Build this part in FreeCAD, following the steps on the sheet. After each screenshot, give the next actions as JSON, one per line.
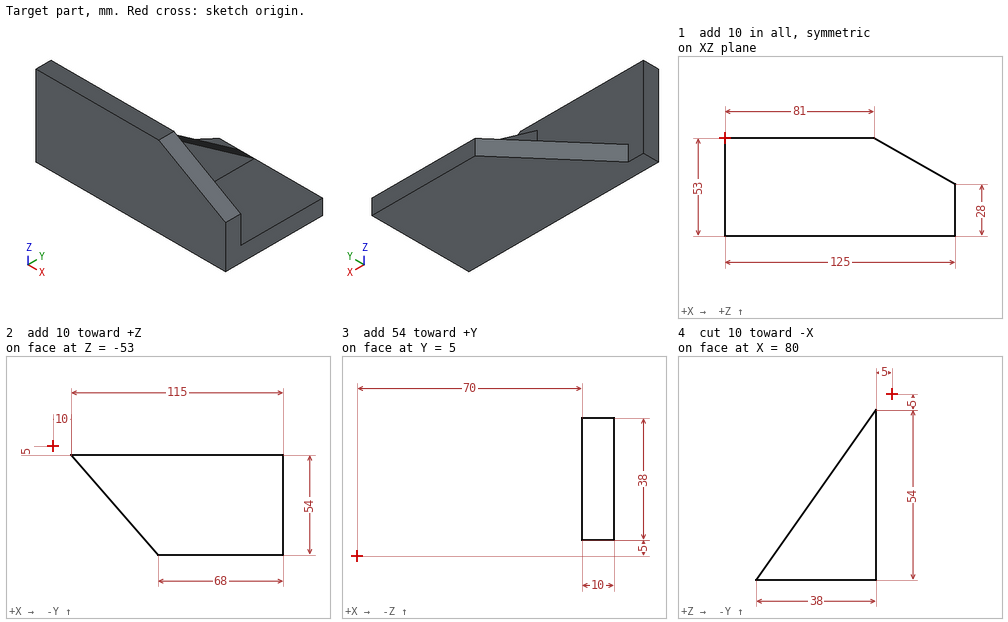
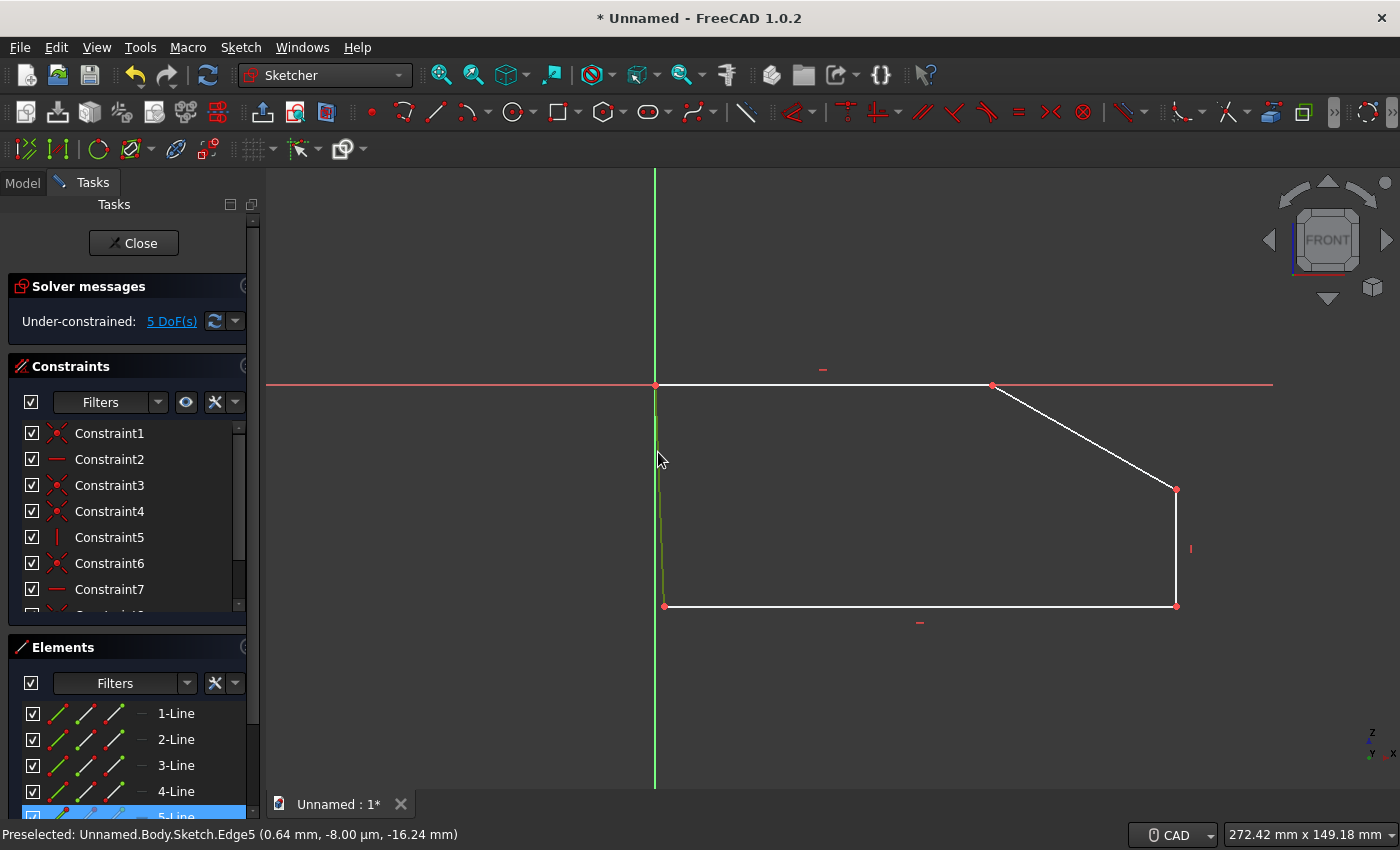
{"action": "key", "text": "v"}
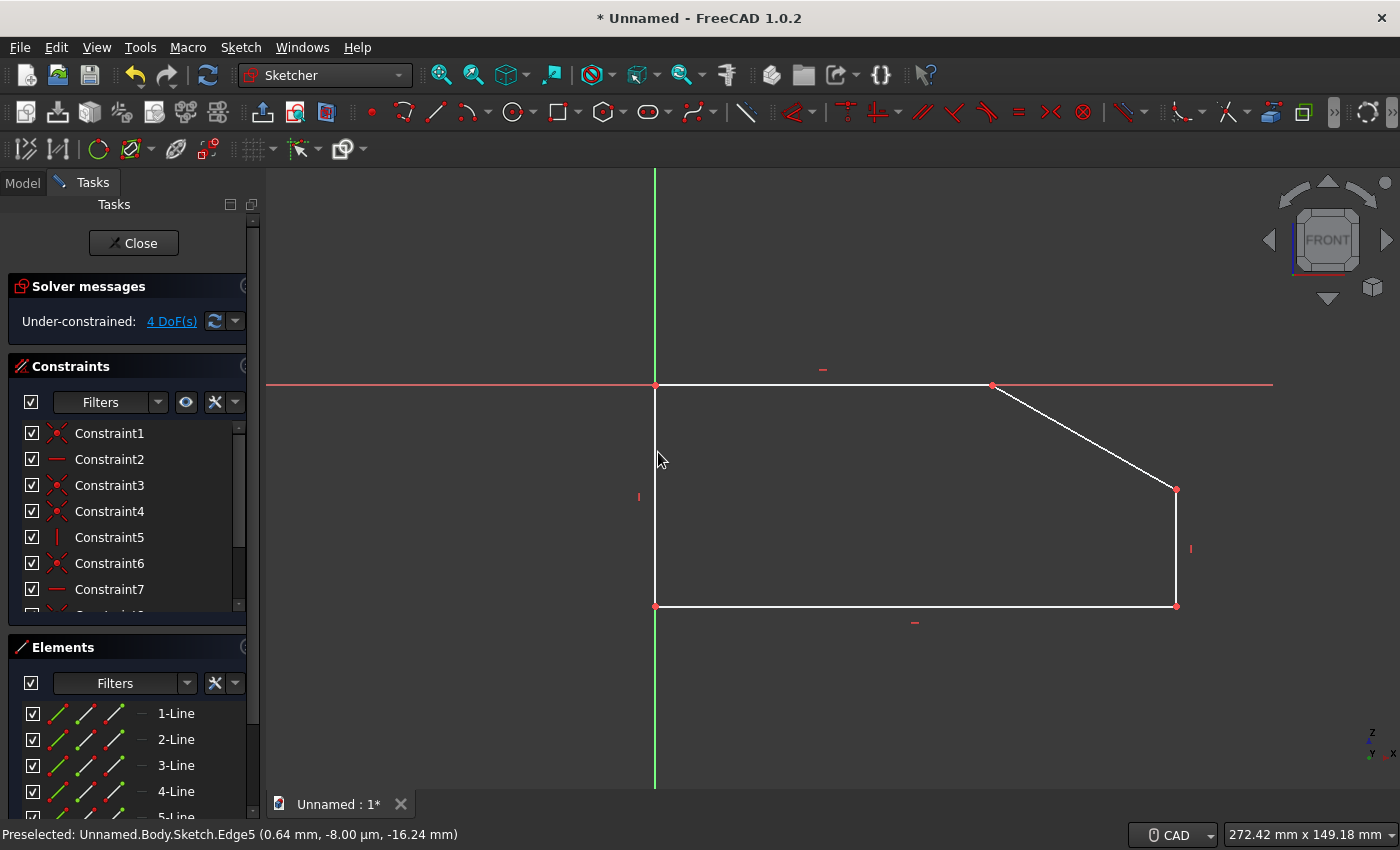
{"action": "left_click", "coordinate": [792, 112]}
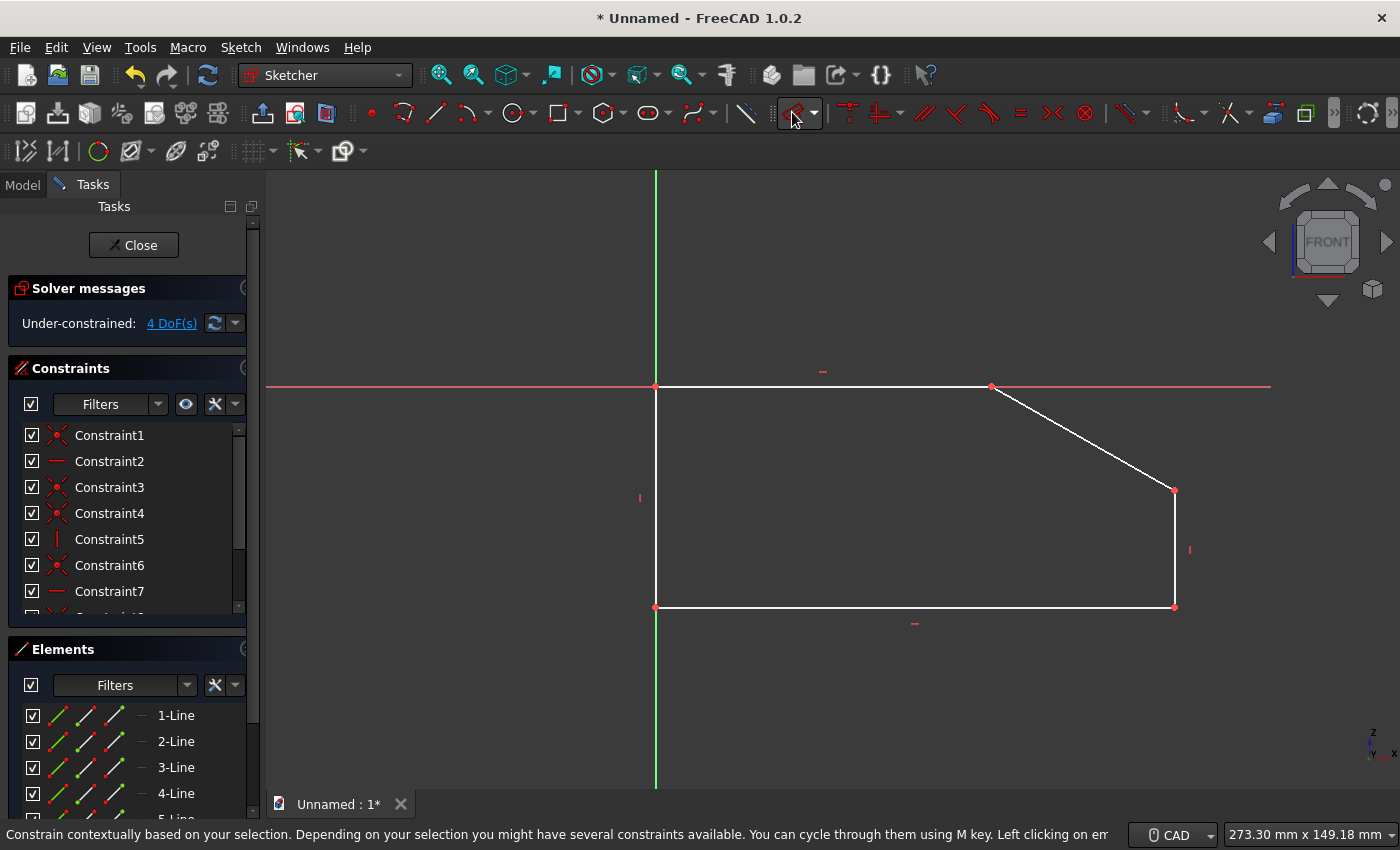
{"action": "left_click", "coordinate": [757, 387]}
{"action": "left_click", "coordinate": [824, 353]}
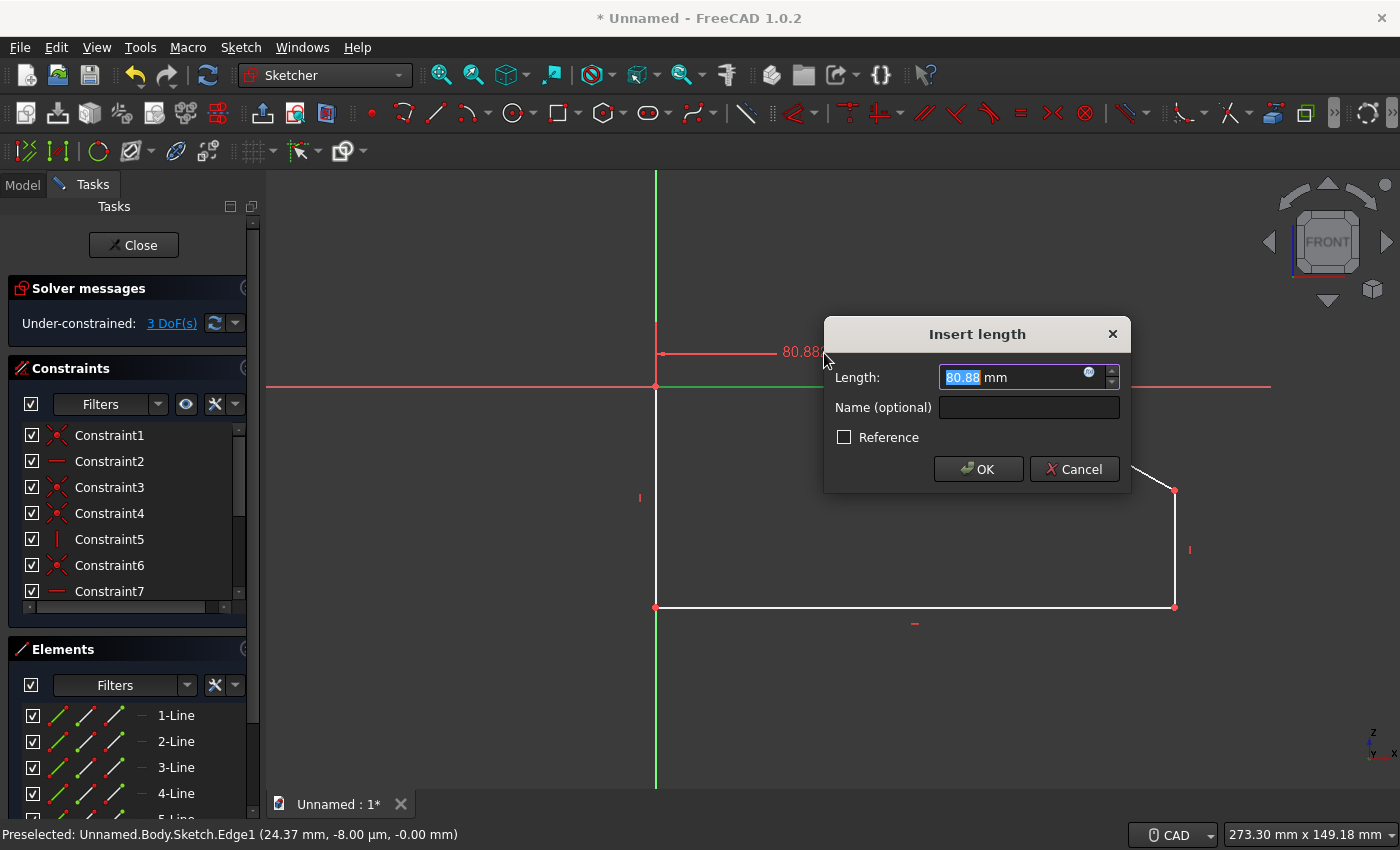
{"action": "type", "text": "81"}
{"action": "key", "text": "Return"}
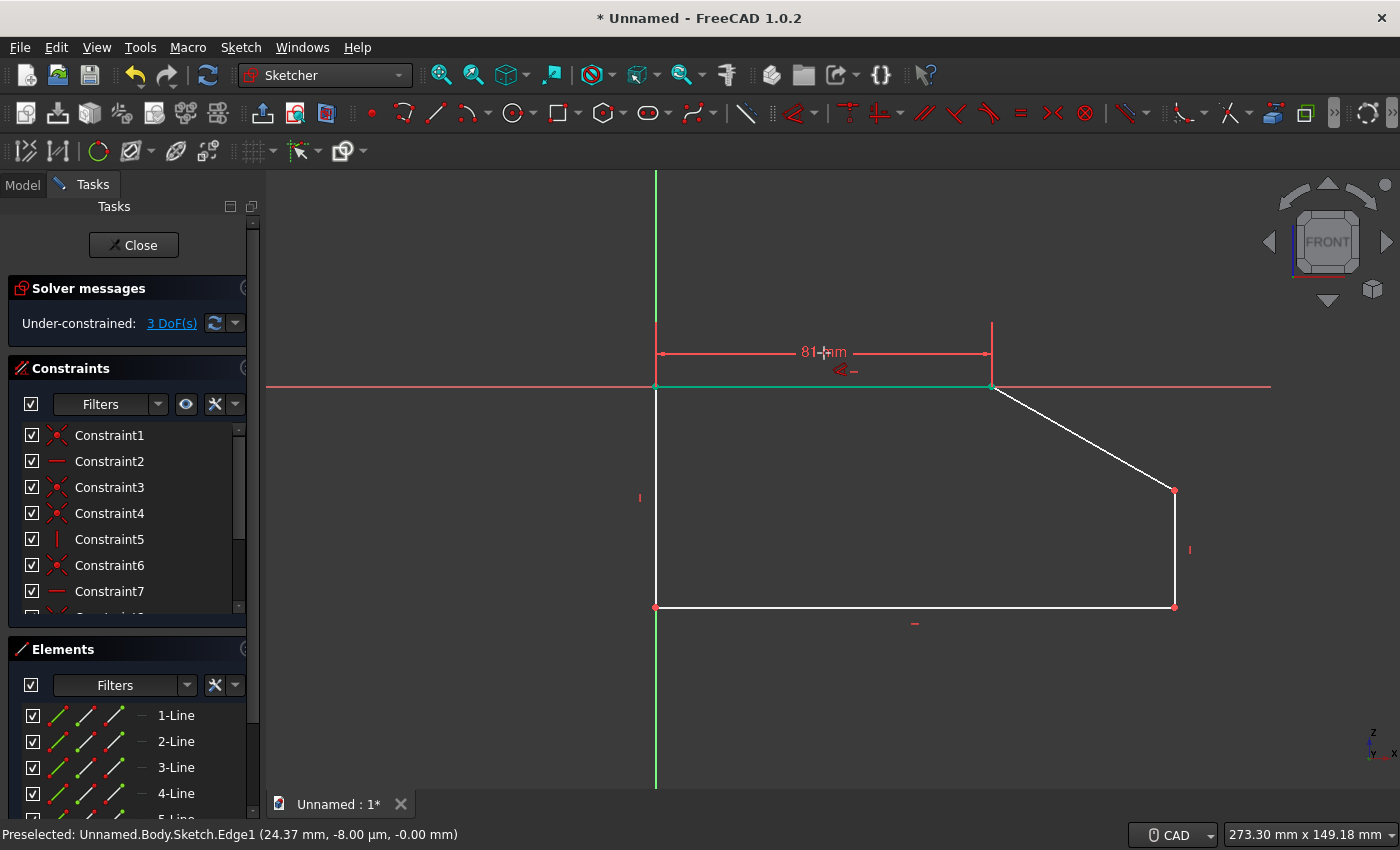
{"action": "left_click", "coordinate": [1175, 526]}
{"action": "left_click", "coordinate": [1209, 549]}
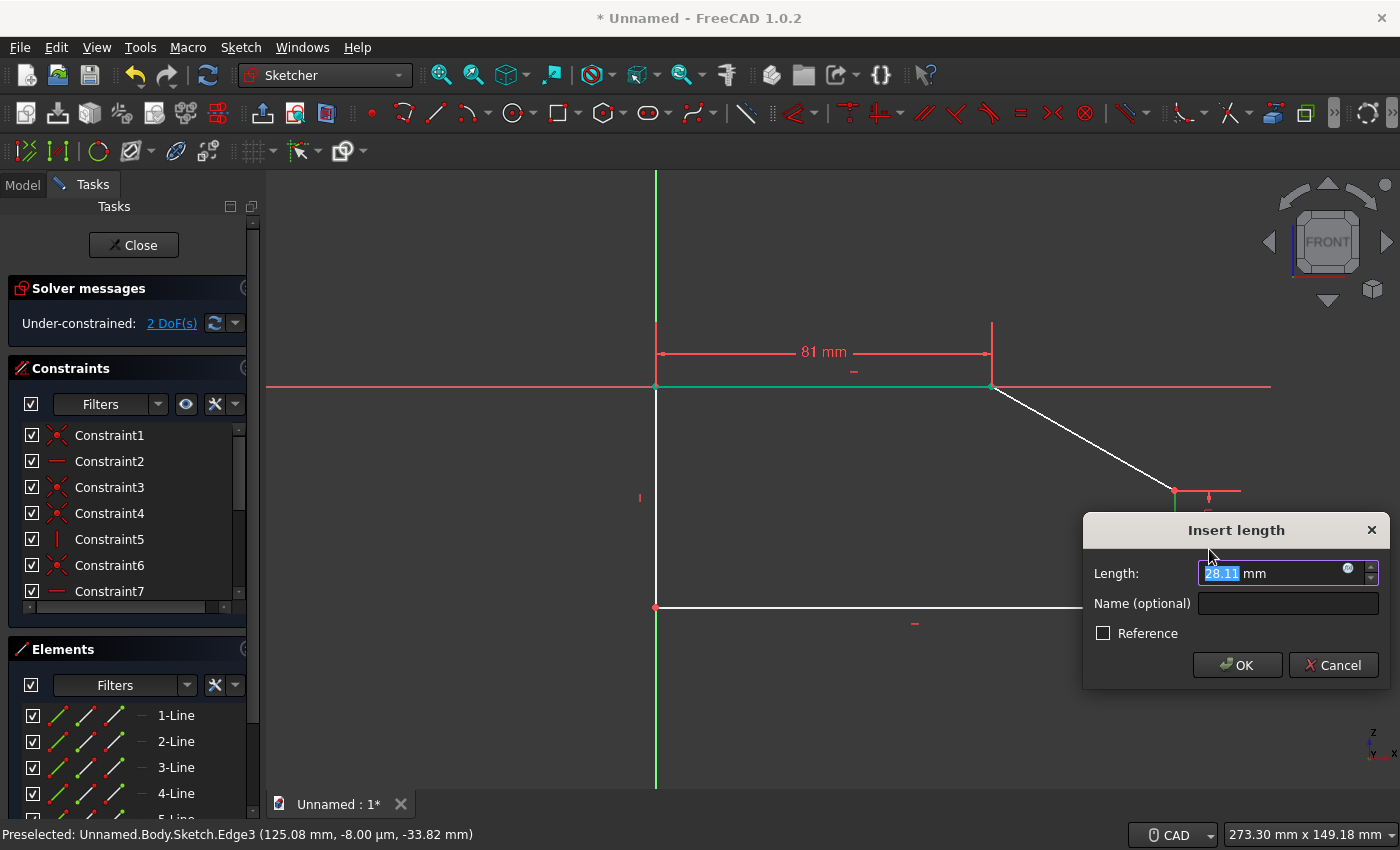
{"action": "type", "text": "28"}
{"action": "key", "text": "Return"}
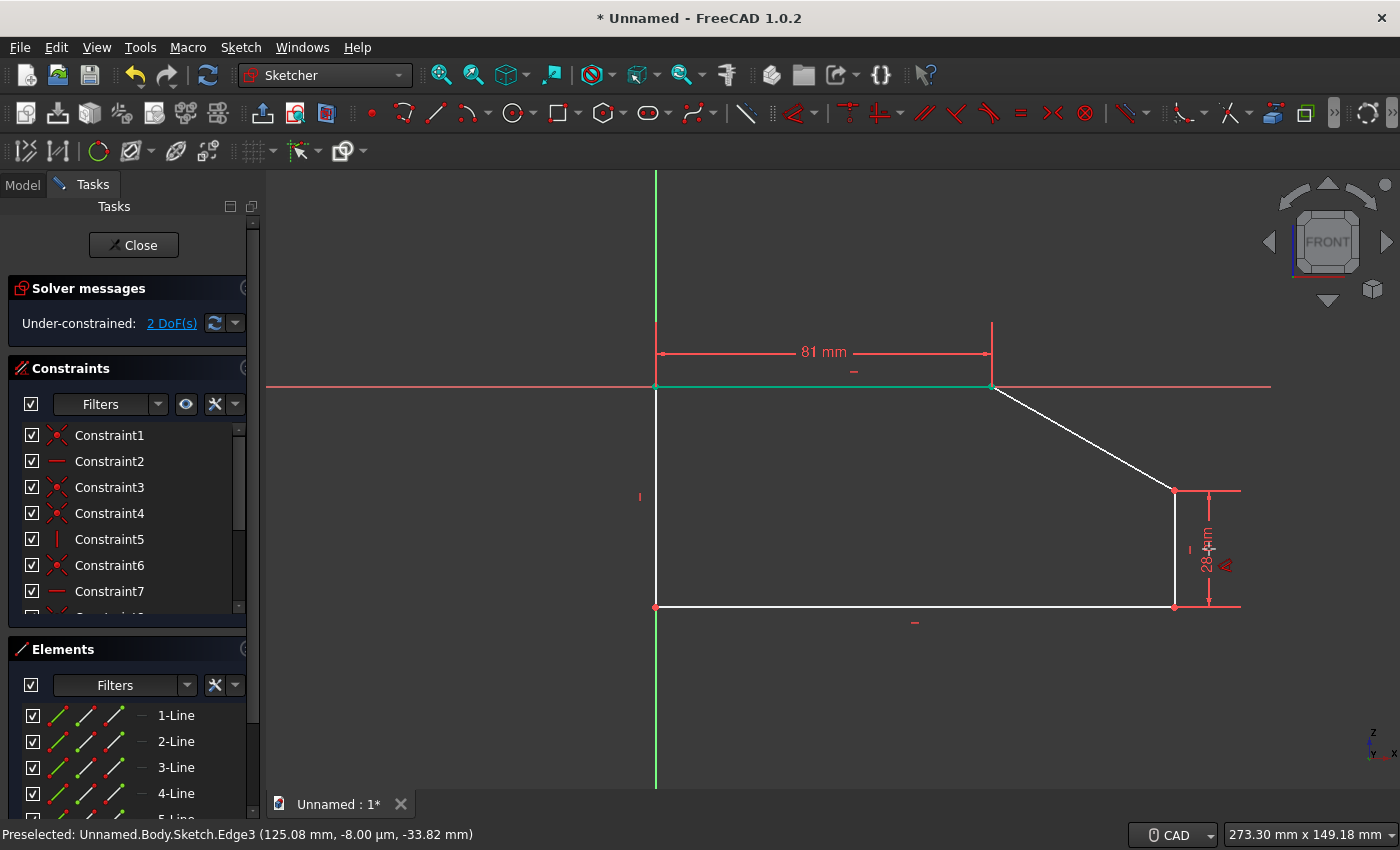
{"action": "left_click", "coordinate": [656, 541]}
{"action": "left_click", "coordinate": [622, 497]}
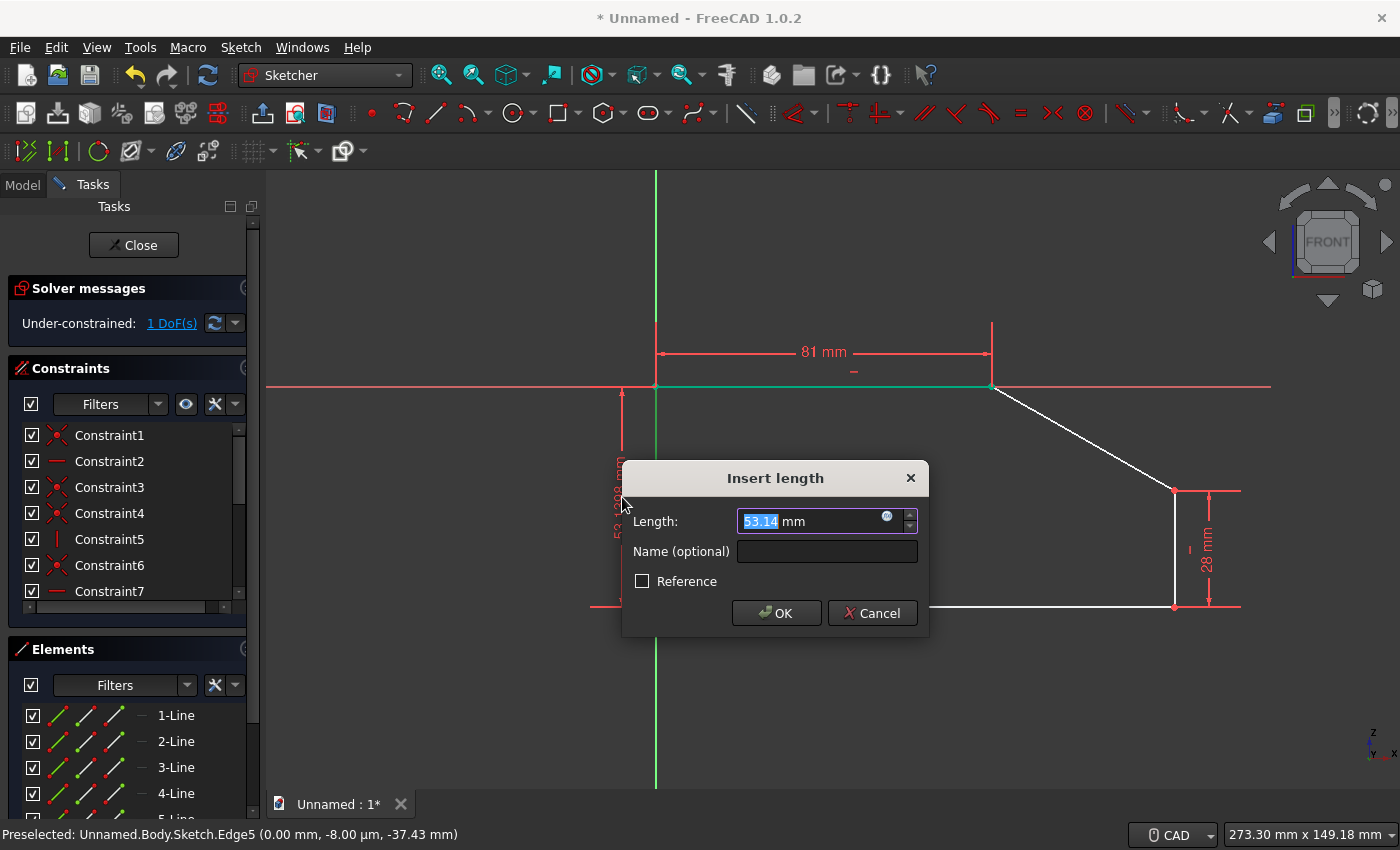
{"action": "type", "text": "53"}
{"action": "key", "text": "Return"}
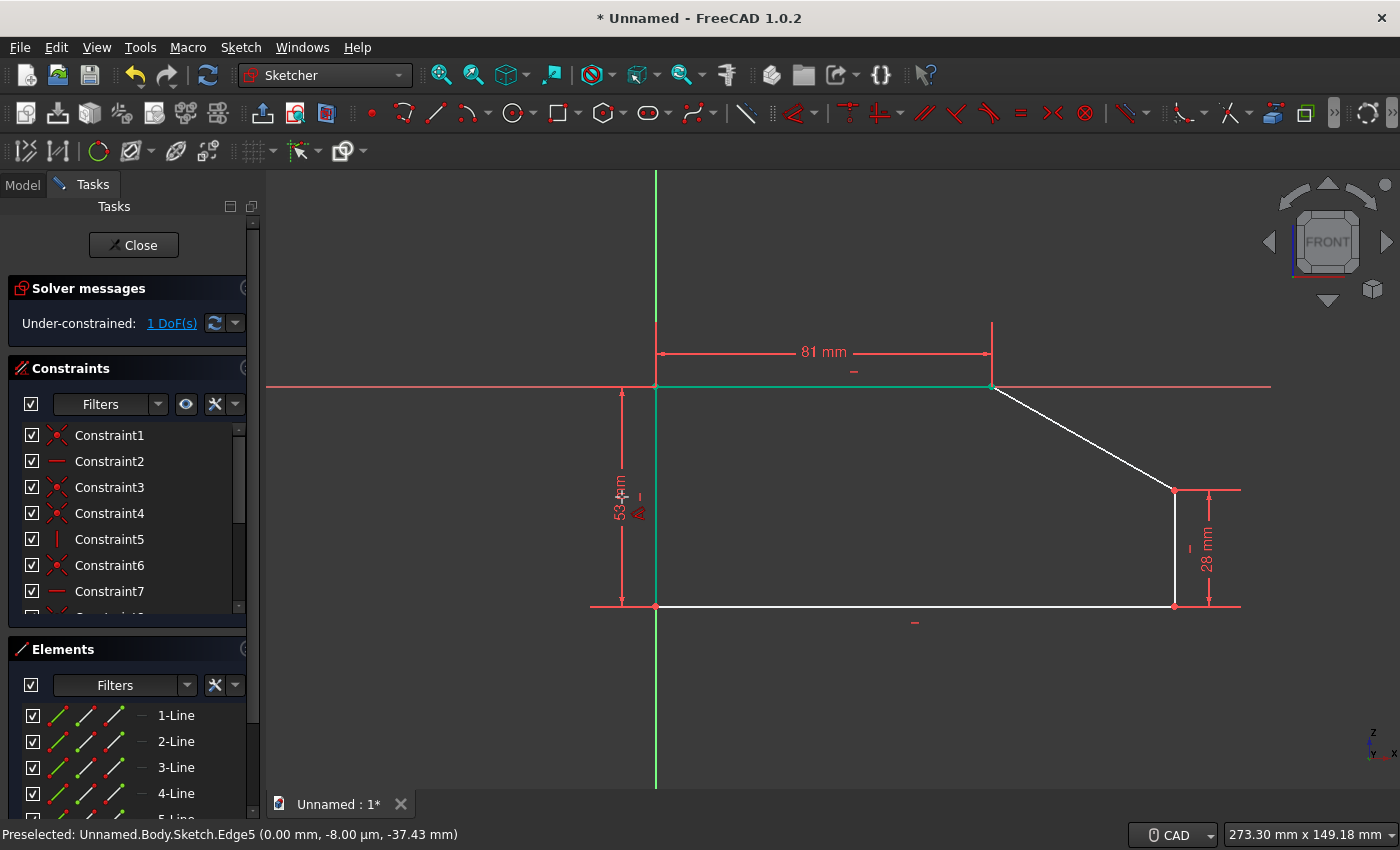
{"action": "left_click", "coordinate": [1019, 607]}
{"action": "left_click", "coordinate": [915, 641]}